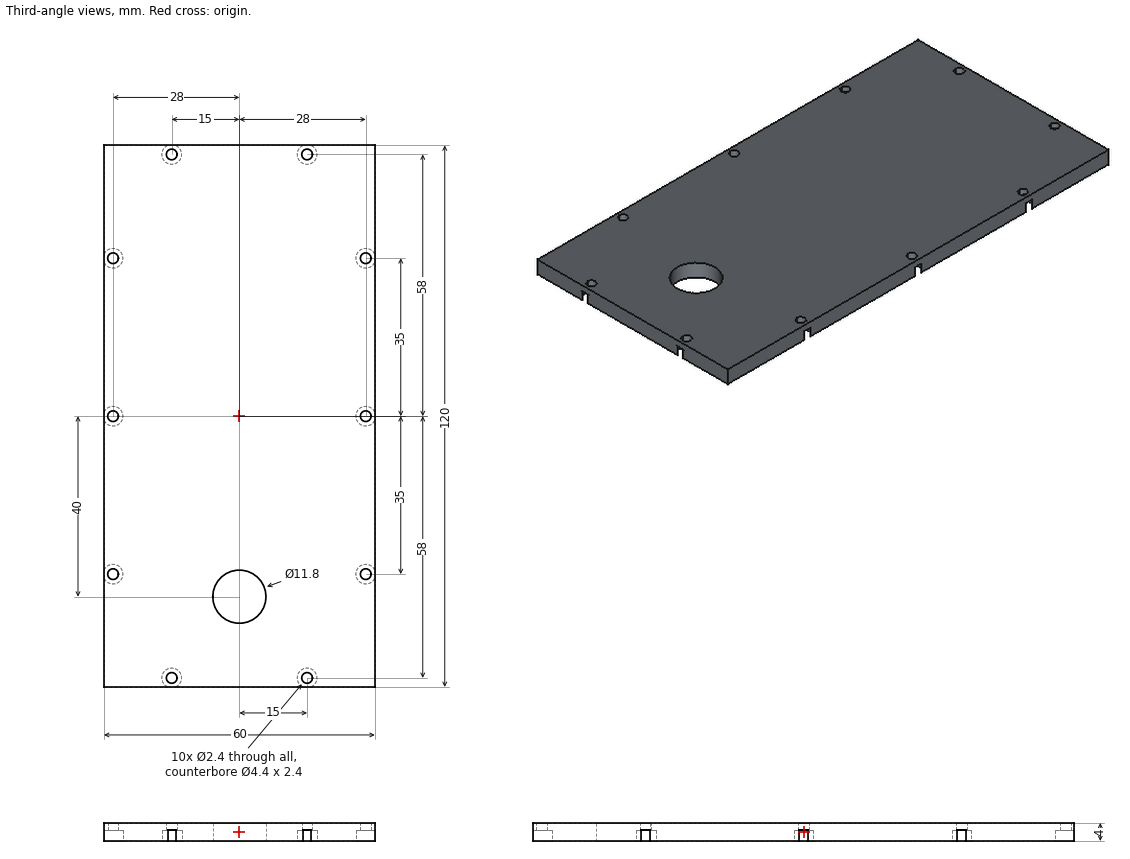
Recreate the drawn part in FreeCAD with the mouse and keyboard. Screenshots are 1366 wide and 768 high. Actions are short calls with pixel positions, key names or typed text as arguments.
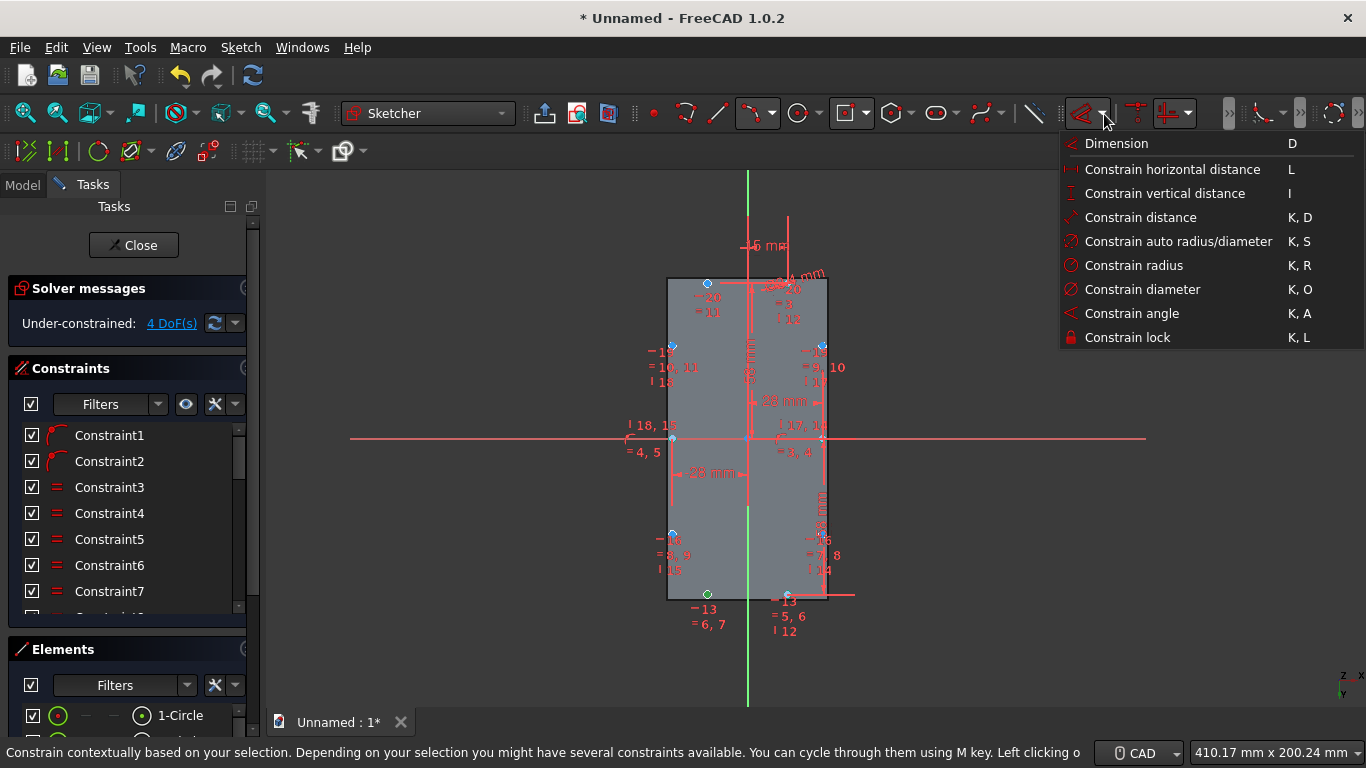
click(1212, 169)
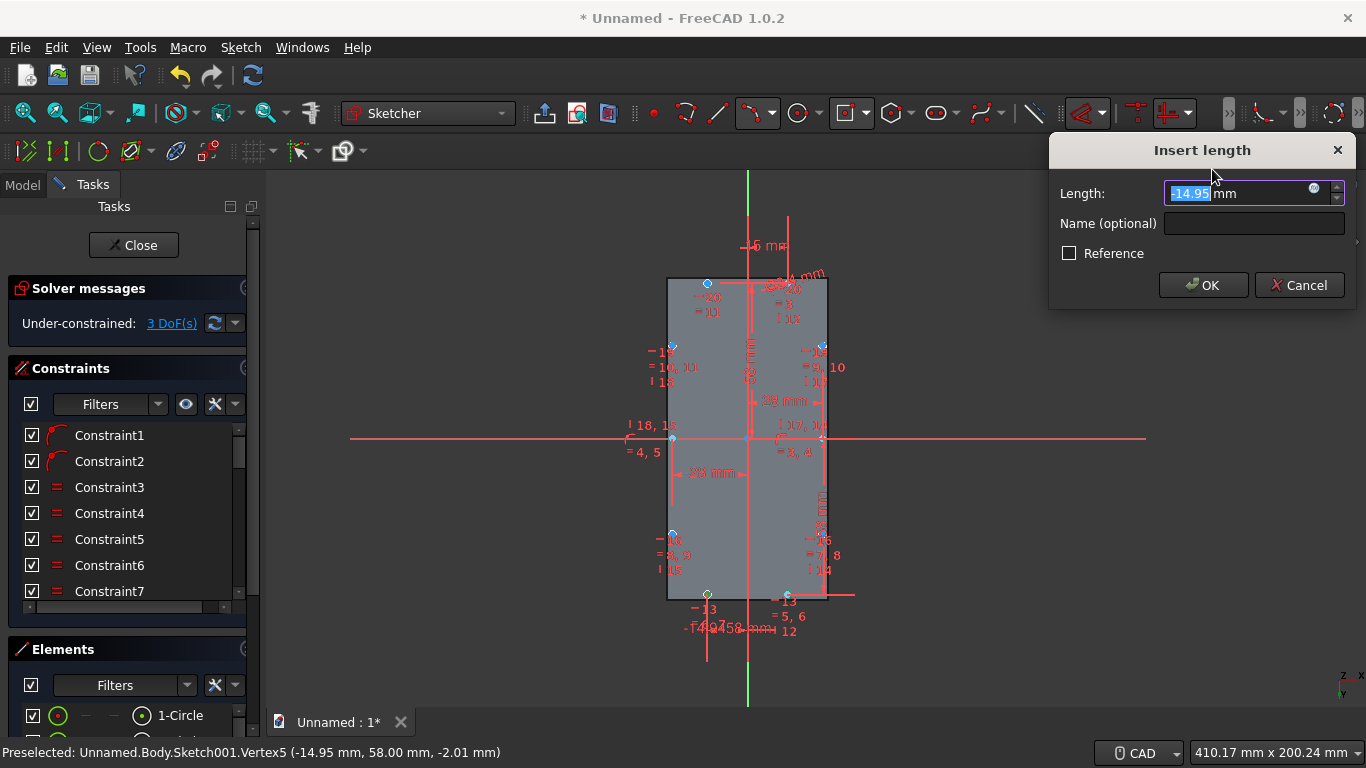
text(-15)
key(Return)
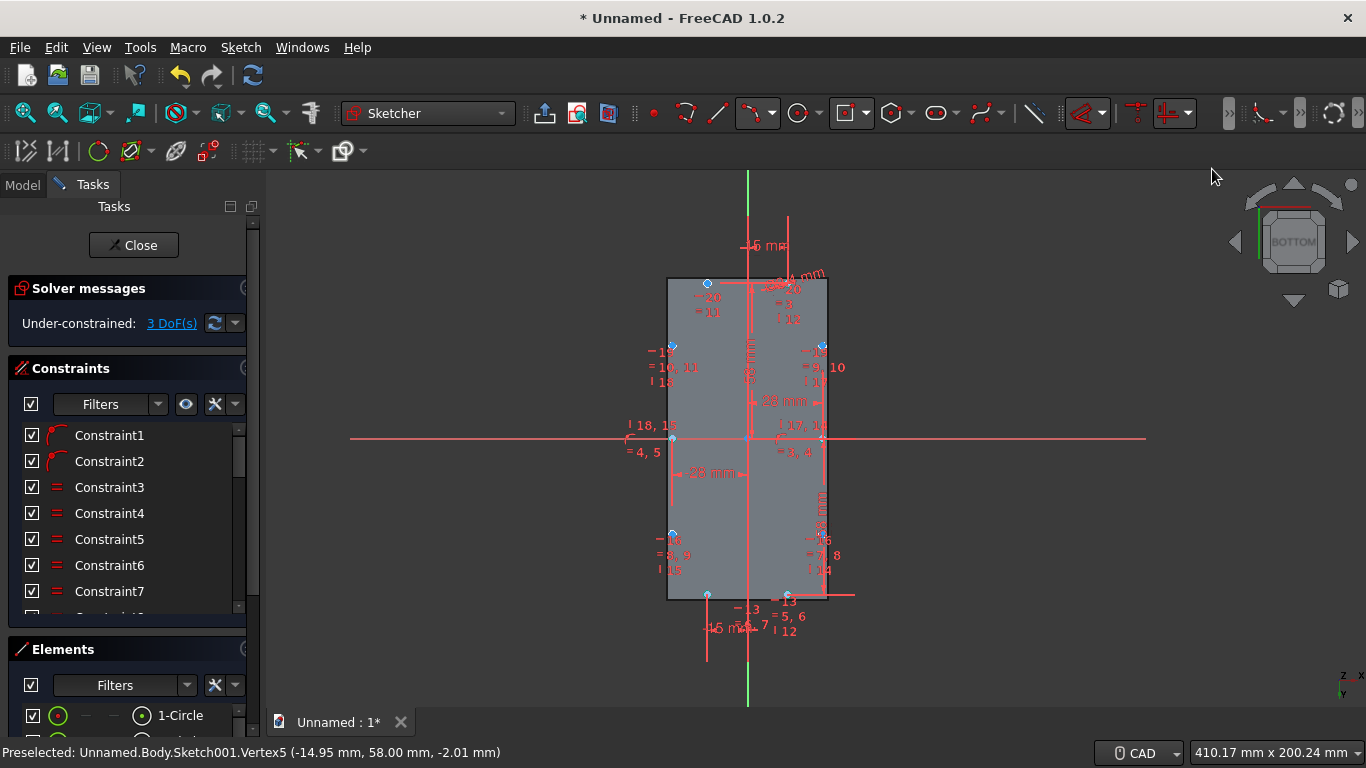
click(823, 534)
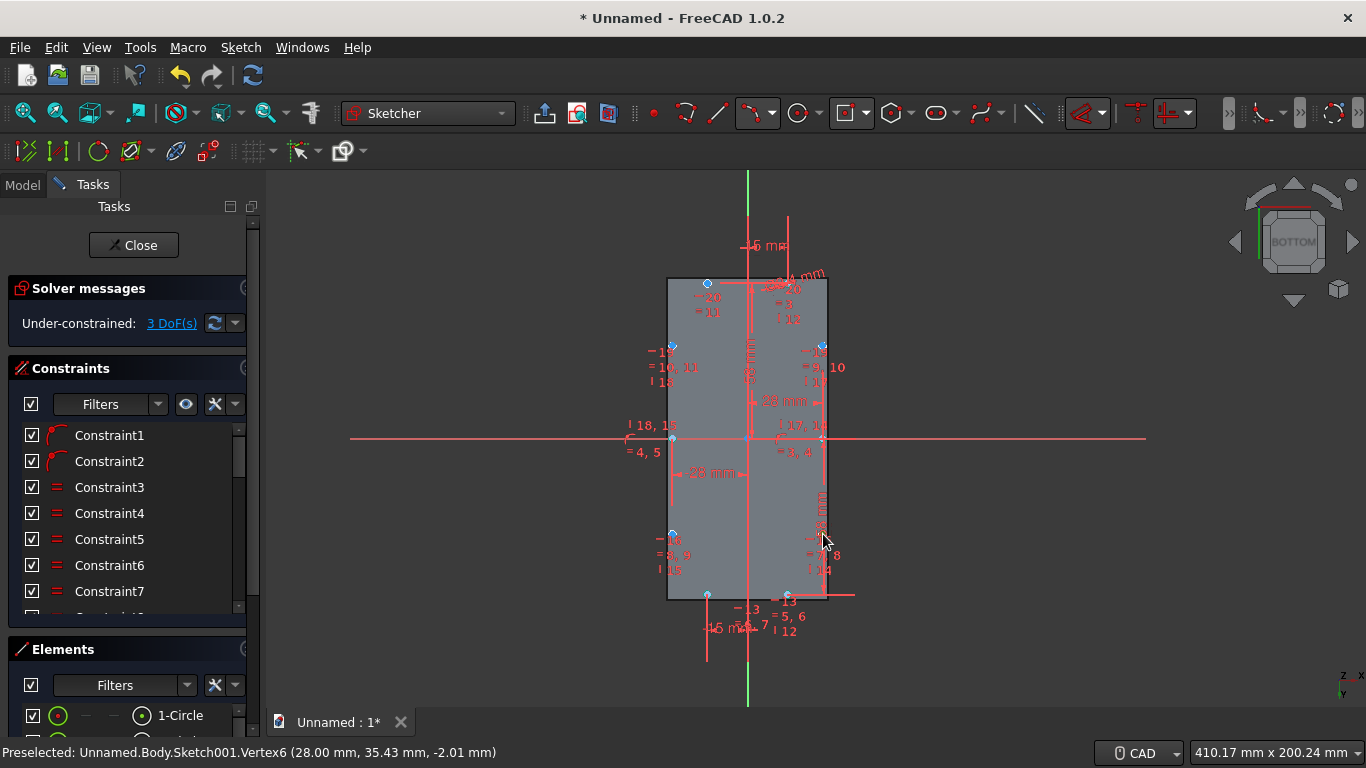
click(1104, 114)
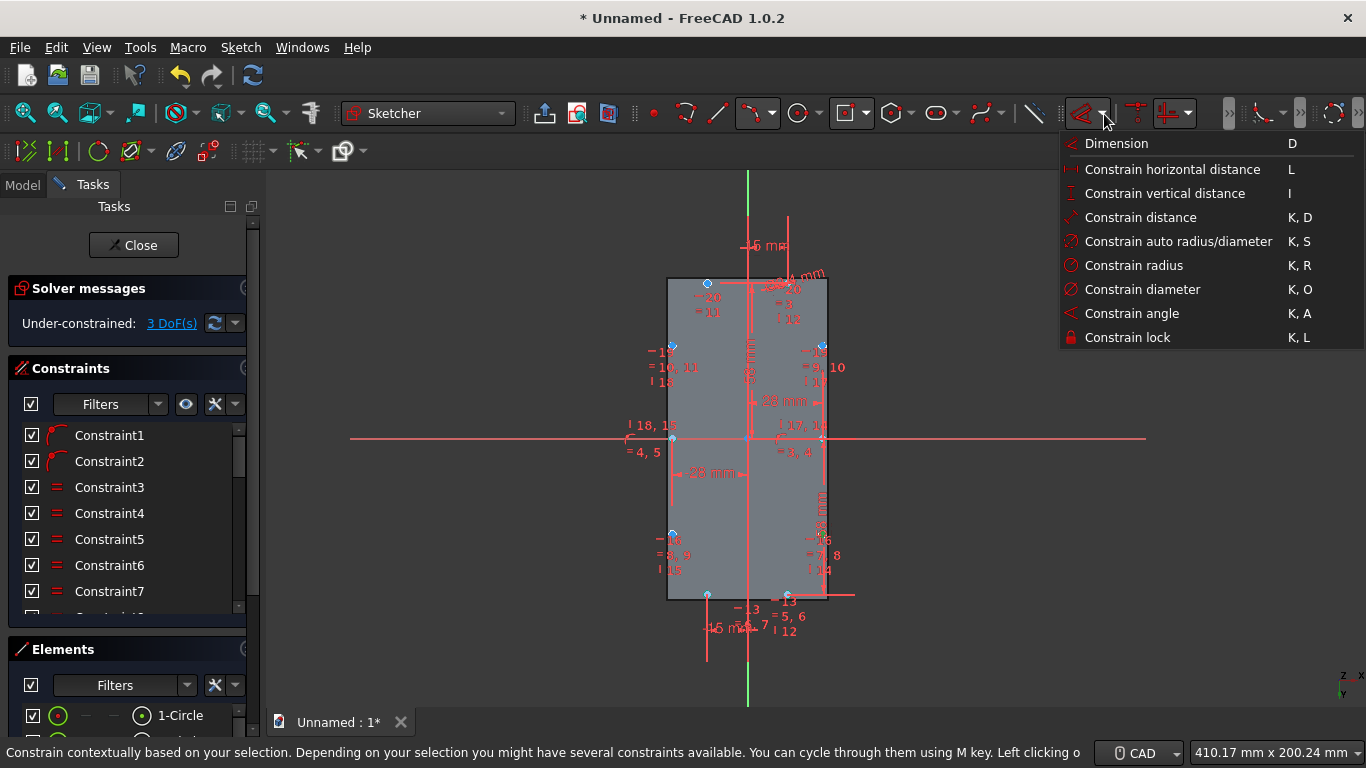
click(1212, 193)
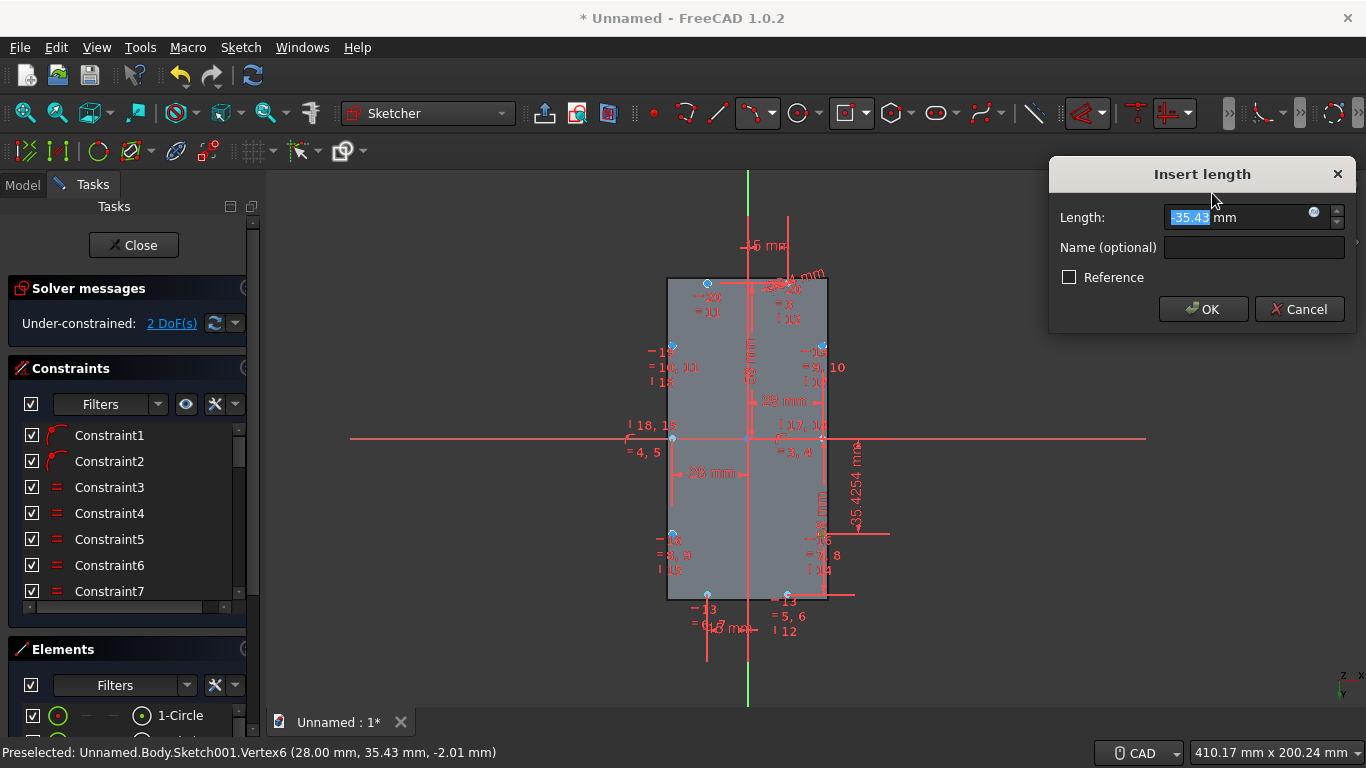
text(-35)
key(Return)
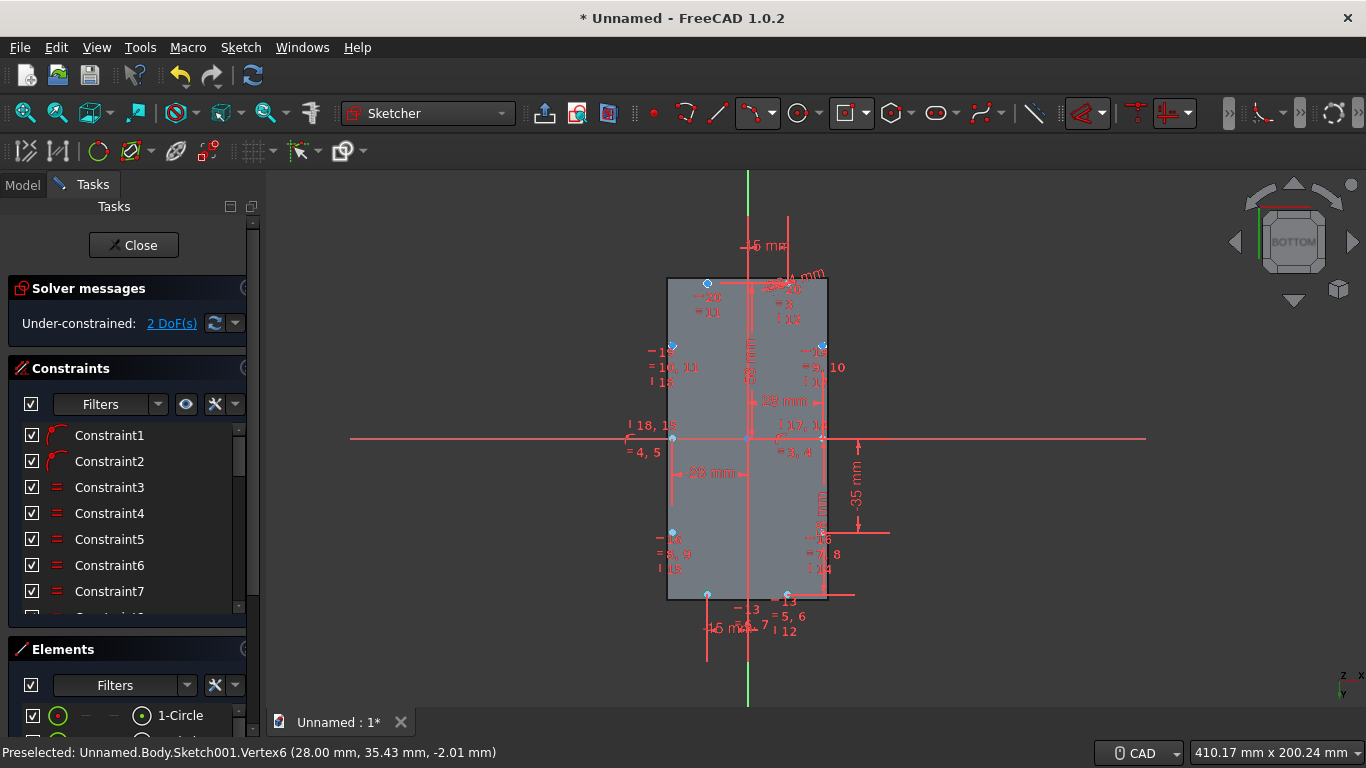
click(823, 346)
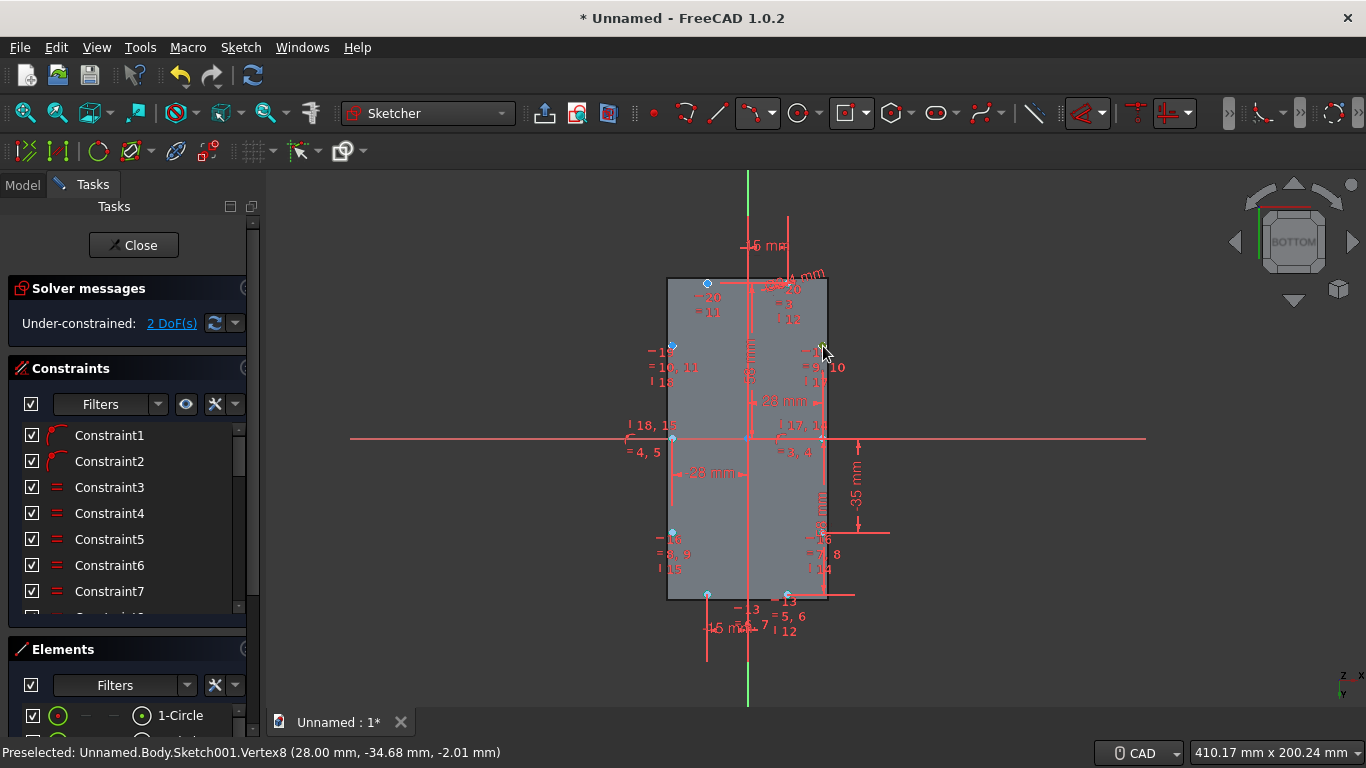
click(1104, 114)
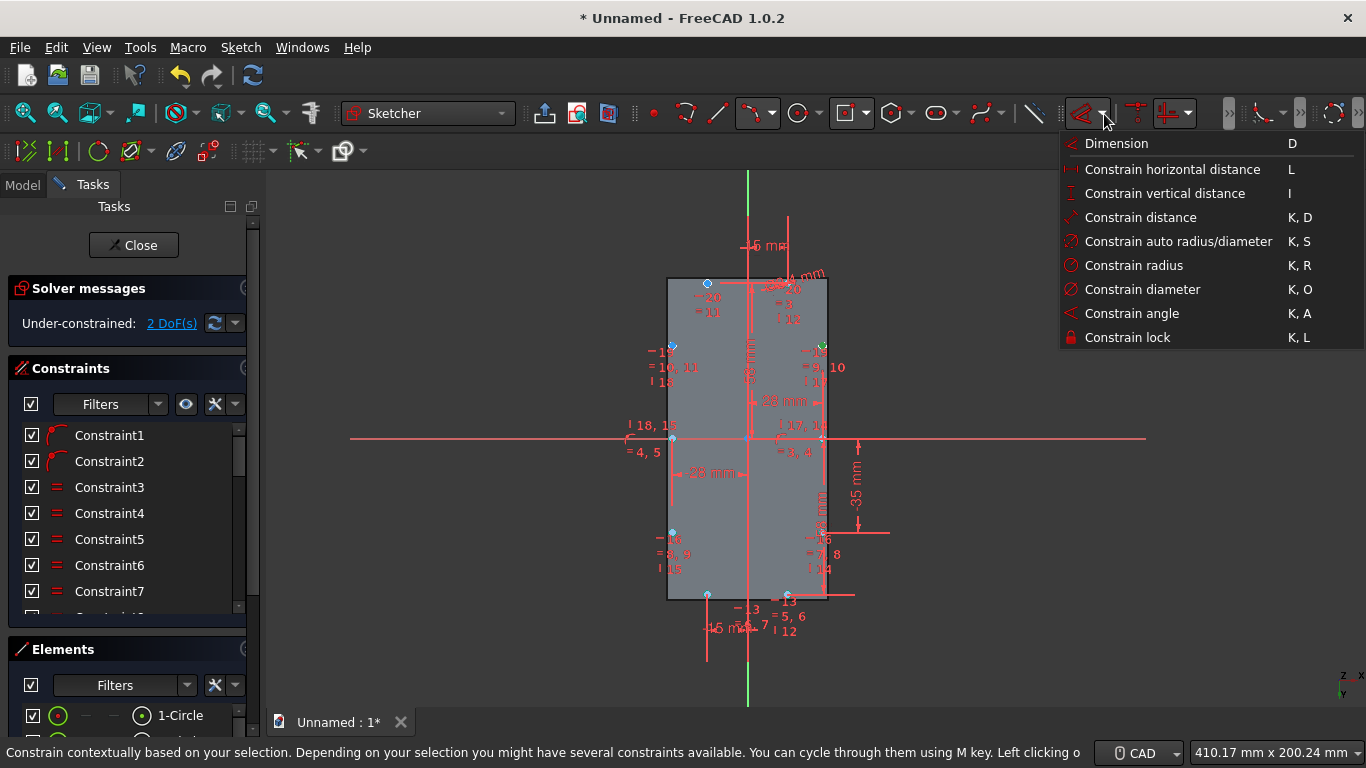
click(1212, 193)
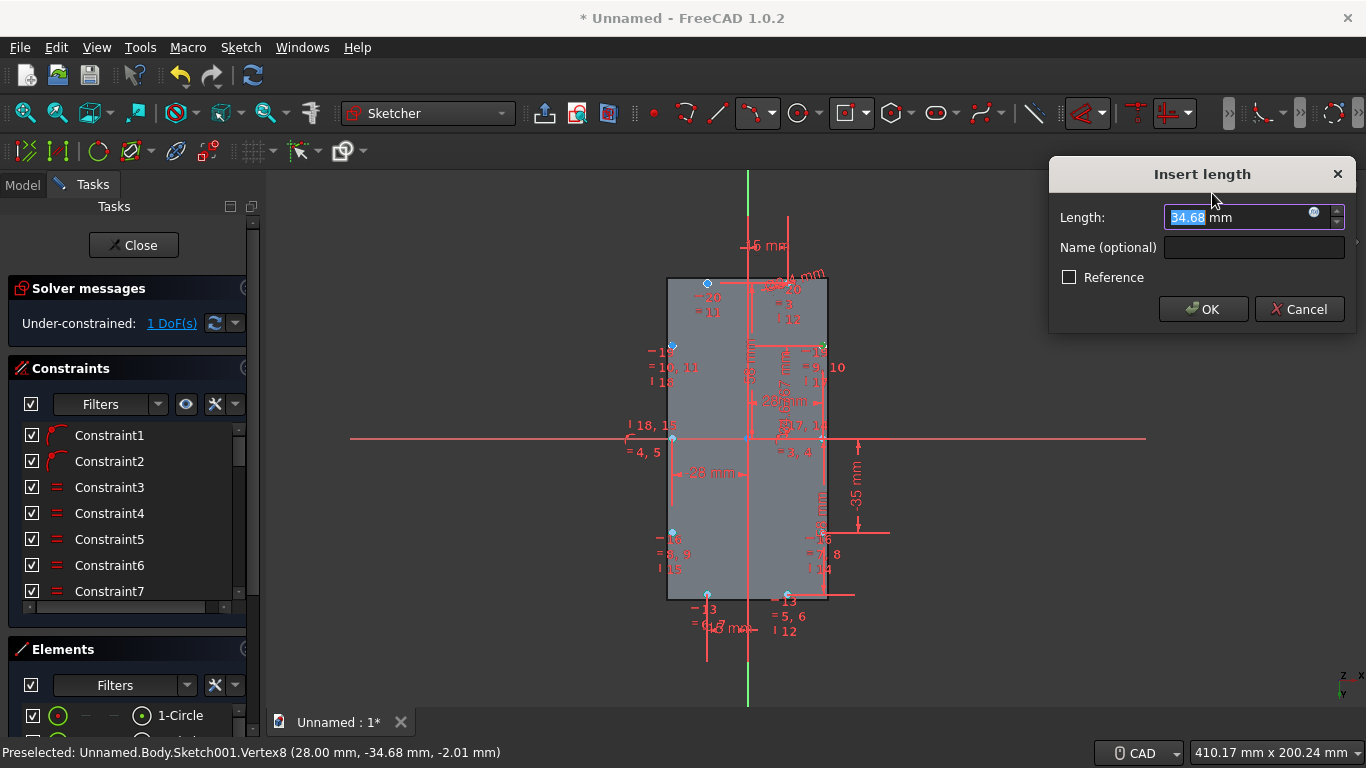
text(35)
key(Return)